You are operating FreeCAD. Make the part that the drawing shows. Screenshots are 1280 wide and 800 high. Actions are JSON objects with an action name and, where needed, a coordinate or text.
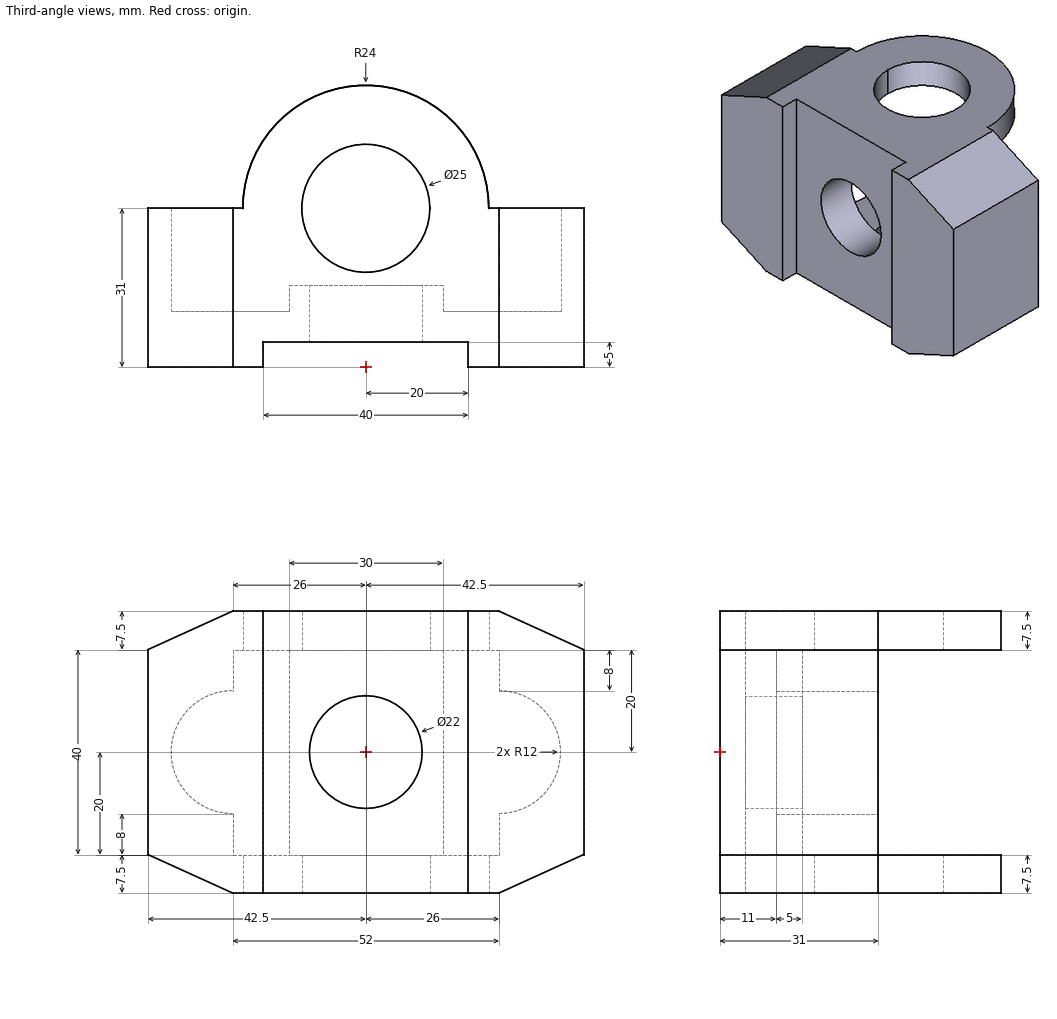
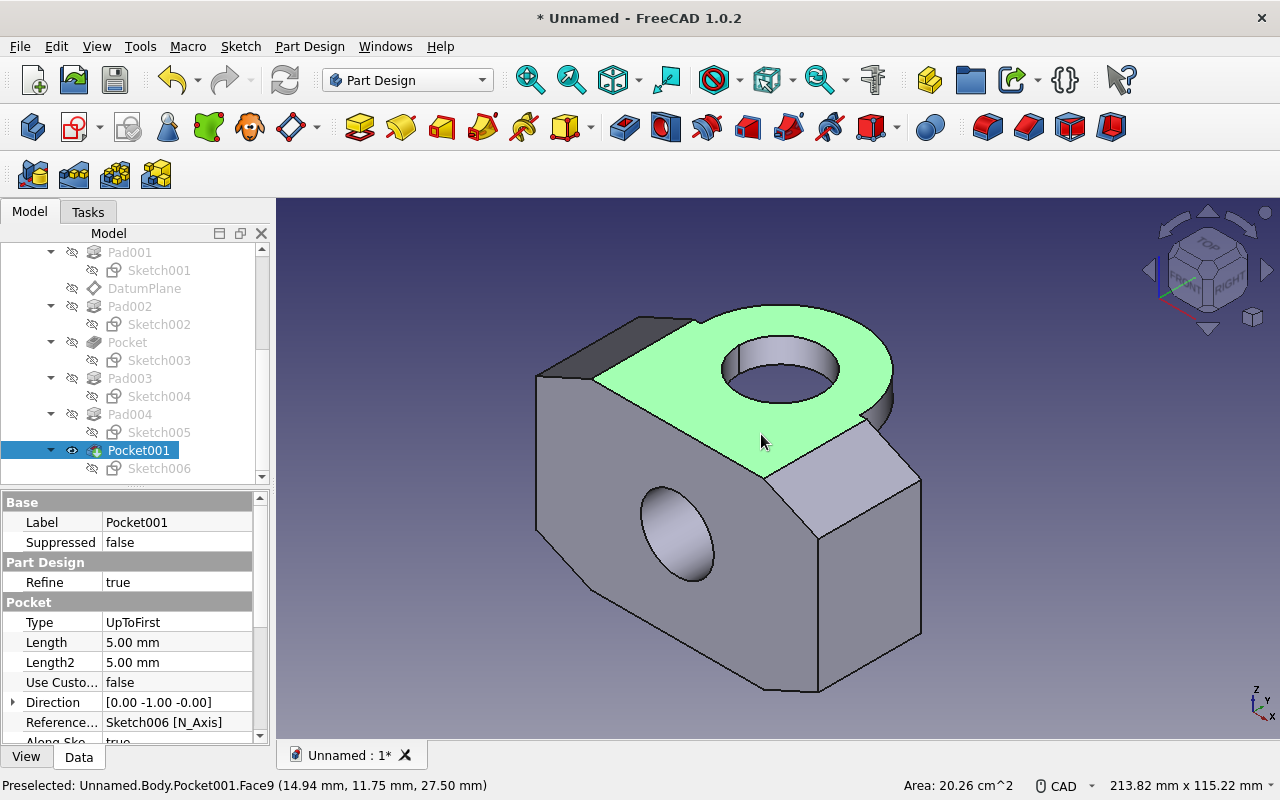
{"action": "left_click", "coordinate": [74, 128]}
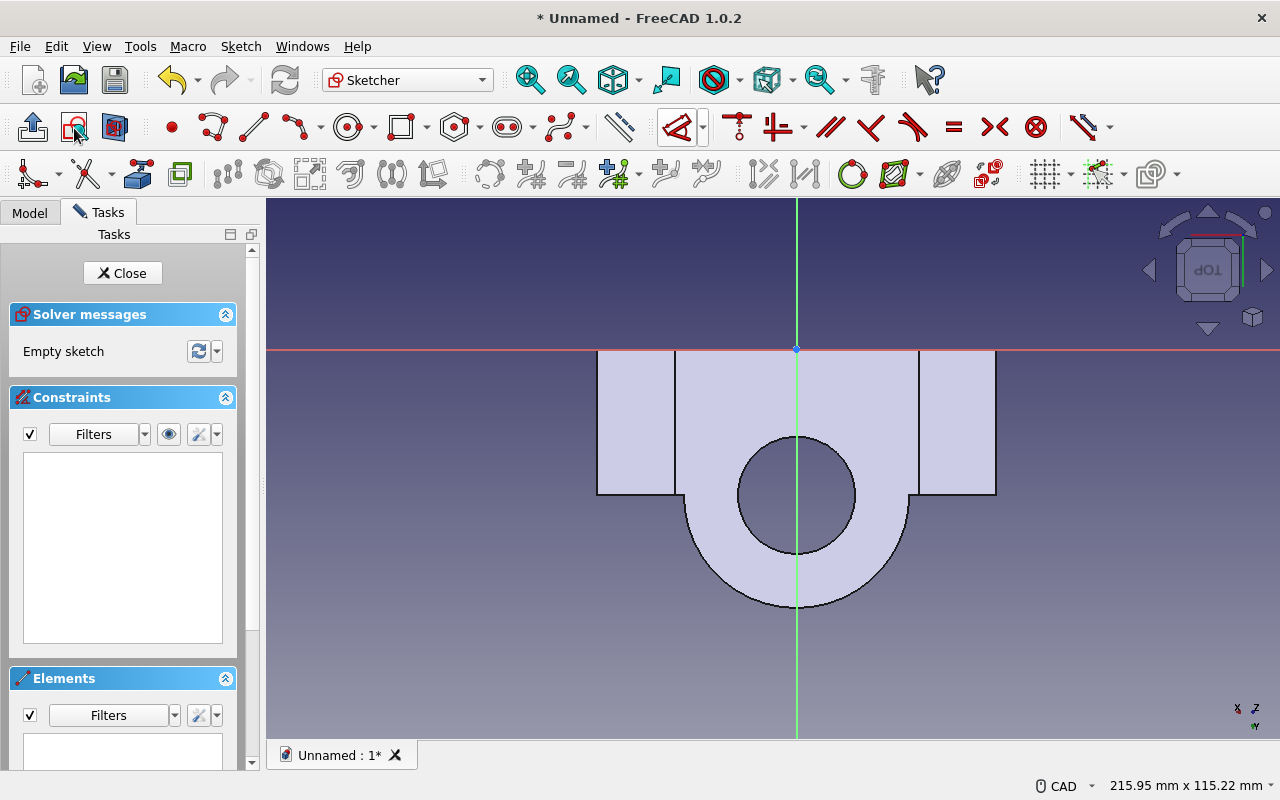
{"action": "scroll", "coordinate": [836, 315], "scroll_direction": "up", "scroll_amount": 6}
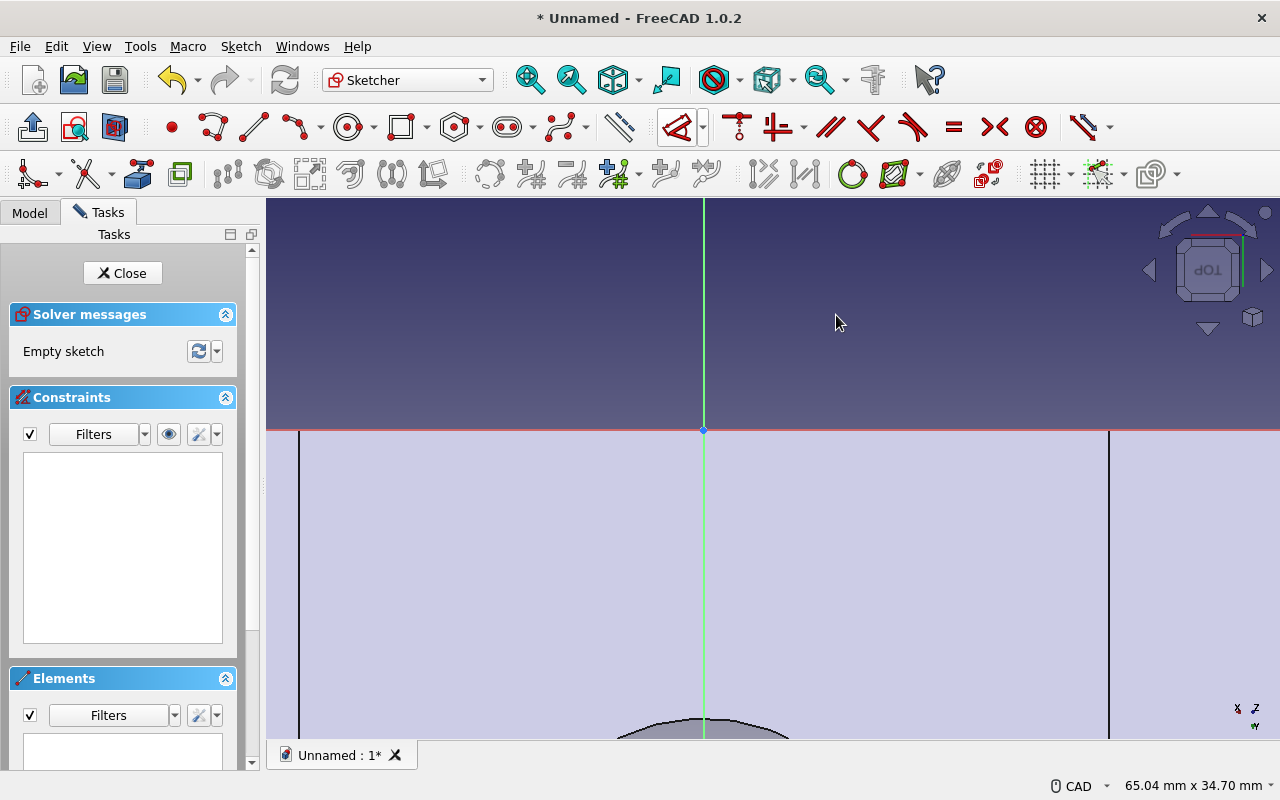
{"action": "left_click", "coordinate": [400, 128]}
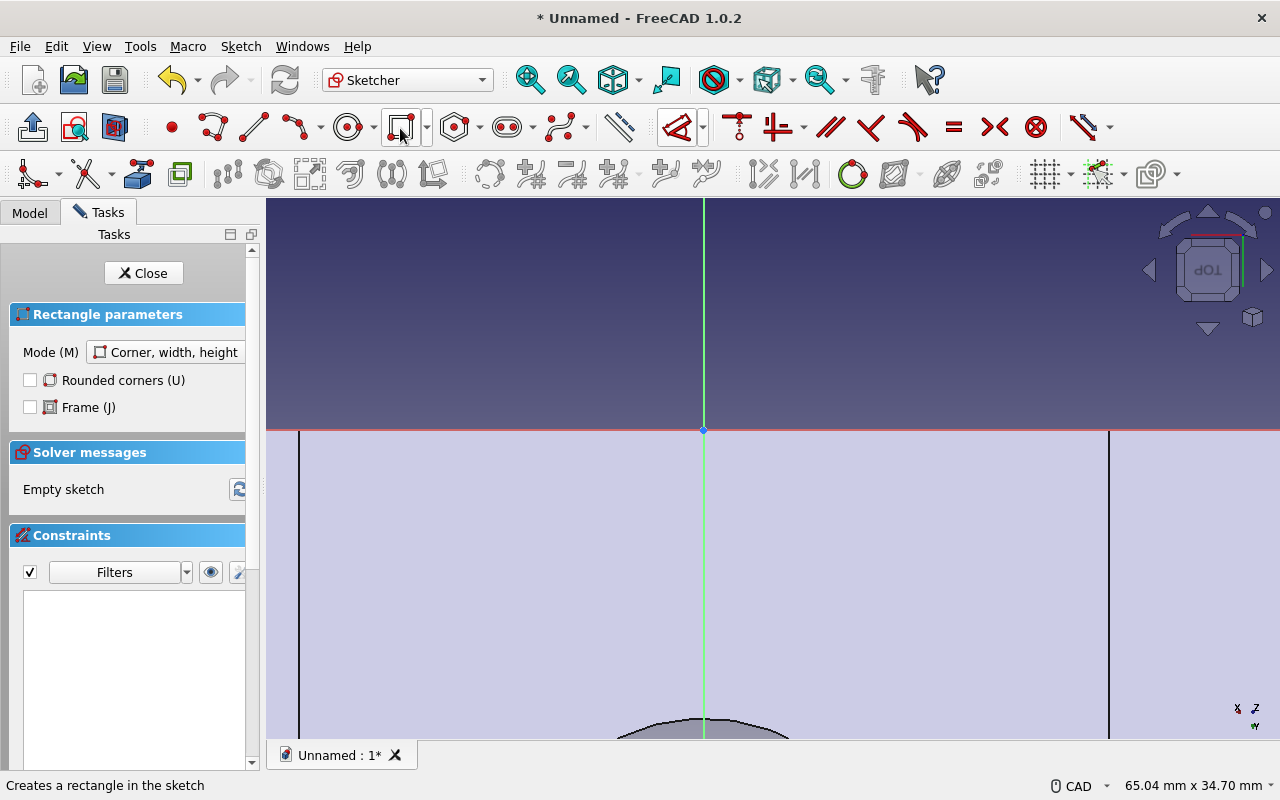
{"action": "left_click", "coordinate": [392, 430]}
{"action": "left_click", "coordinate": [1016, 508]}
{"action": "key", "text": "Escape"}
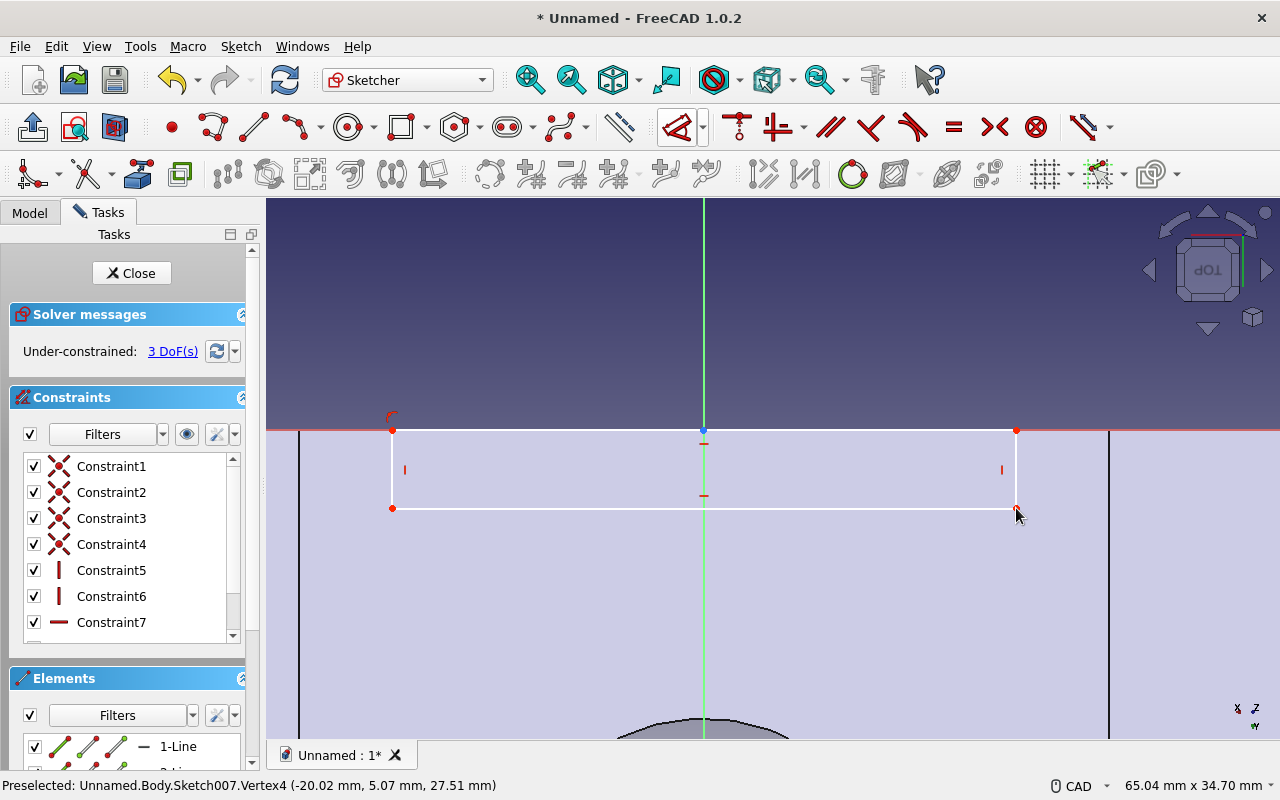
{"action": "left_click", "coordinate": [392, 454]}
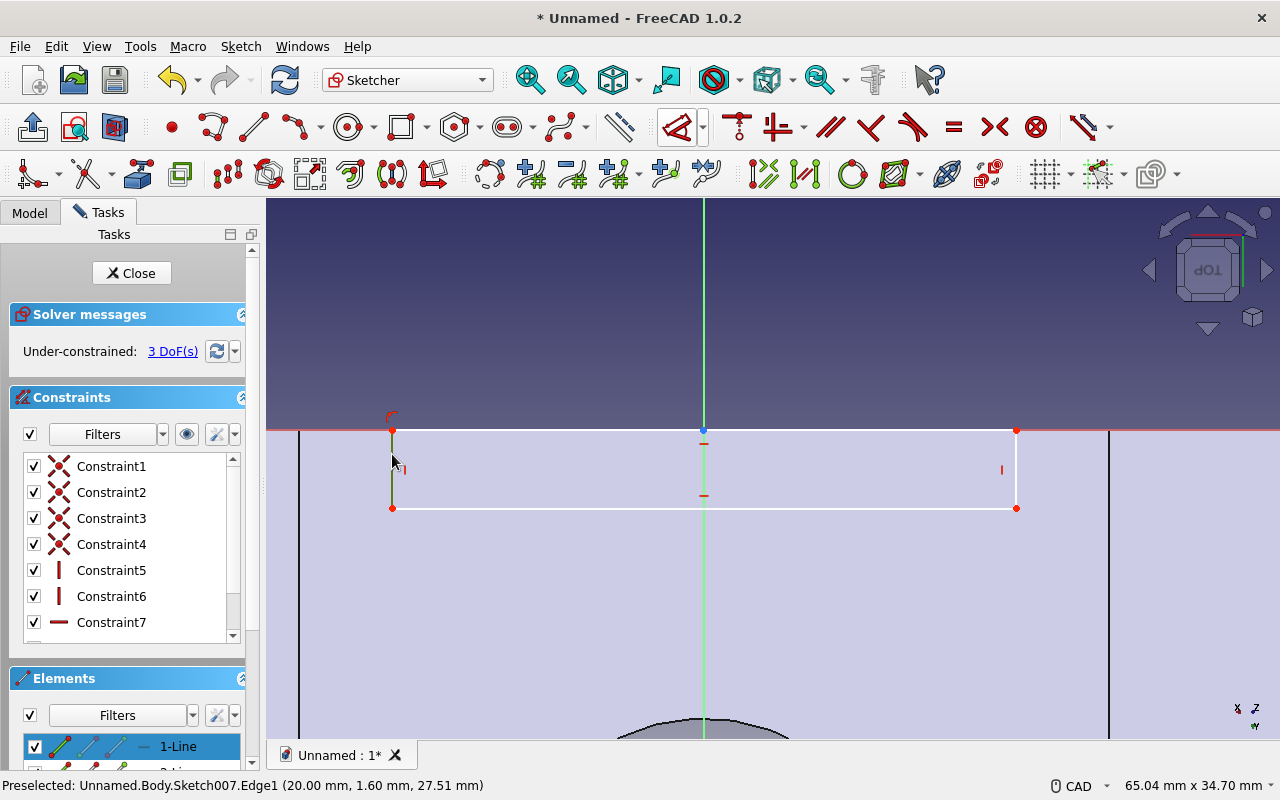
{"action": "key", "text": "i"}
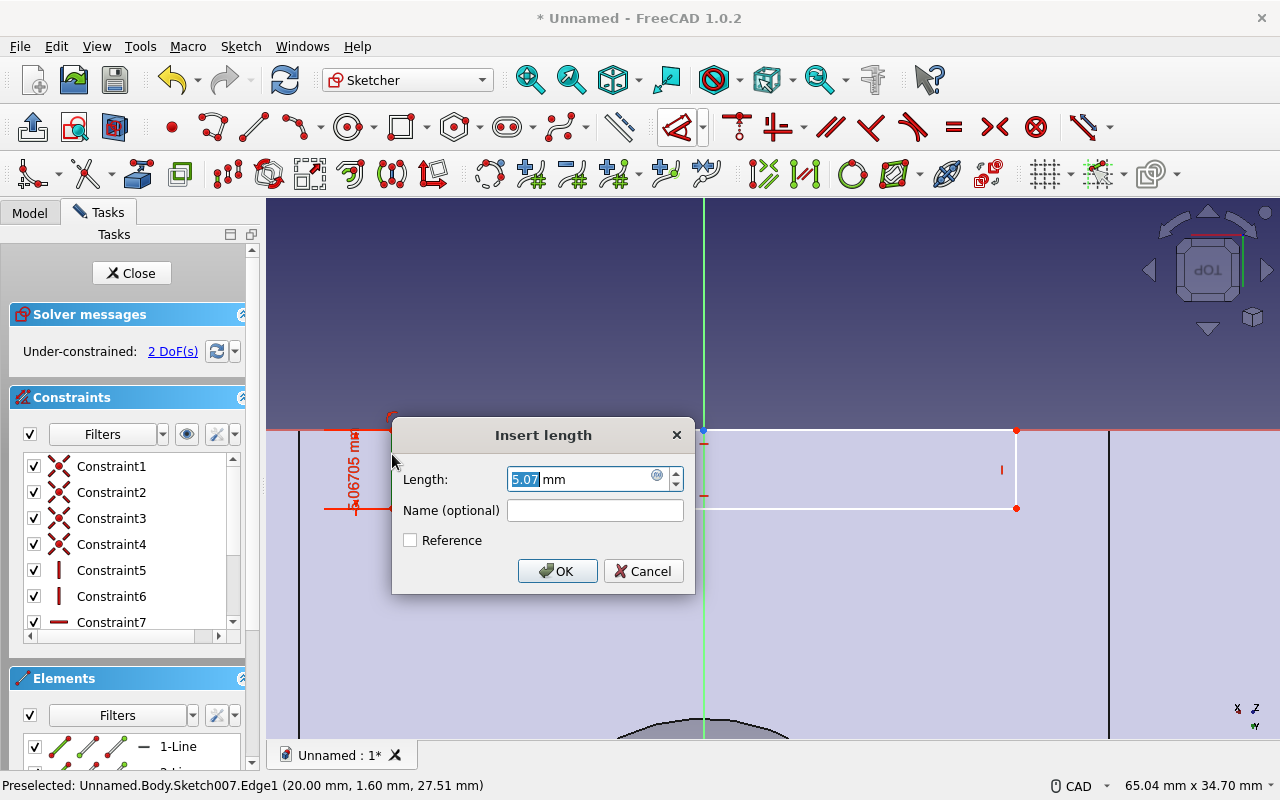
{"action": "type", "text": "5"}
{"action": "key", "text": "Return"}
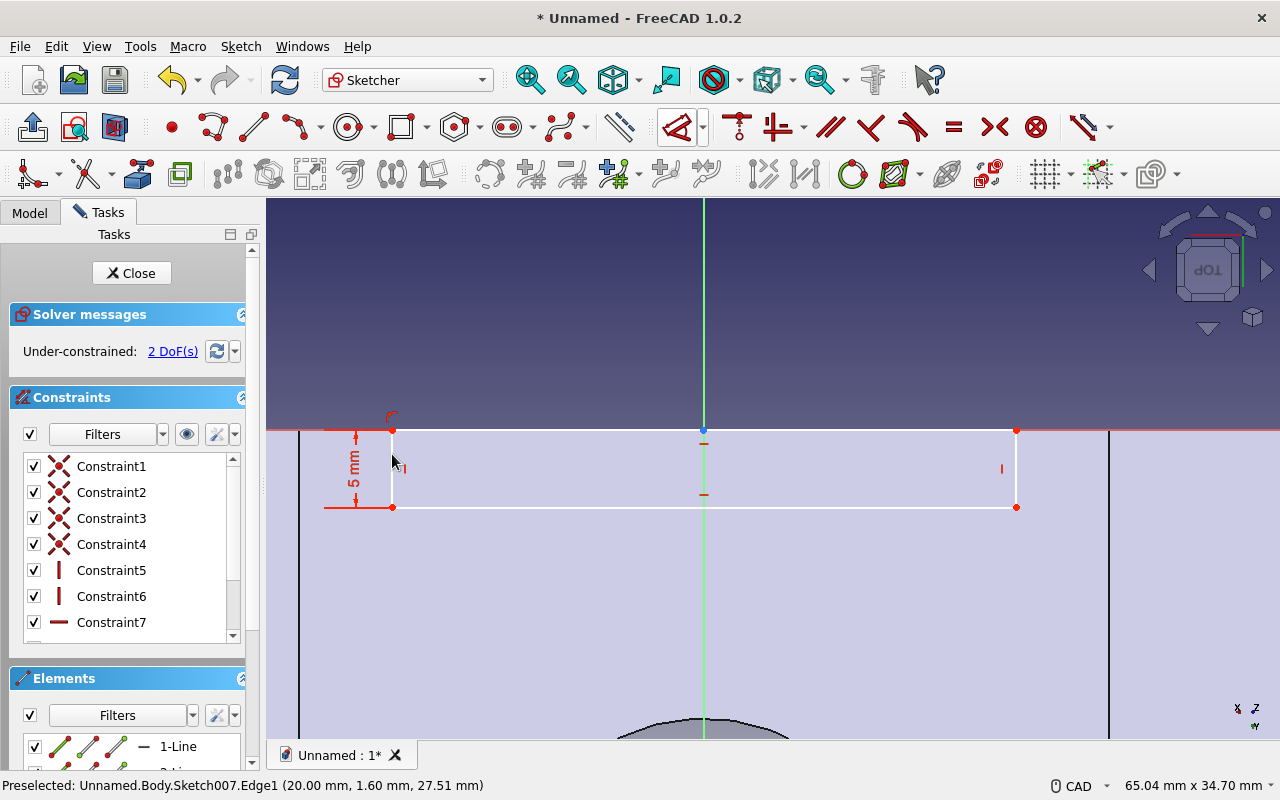
{"action": "left_click", "coordinate": [579, 508]}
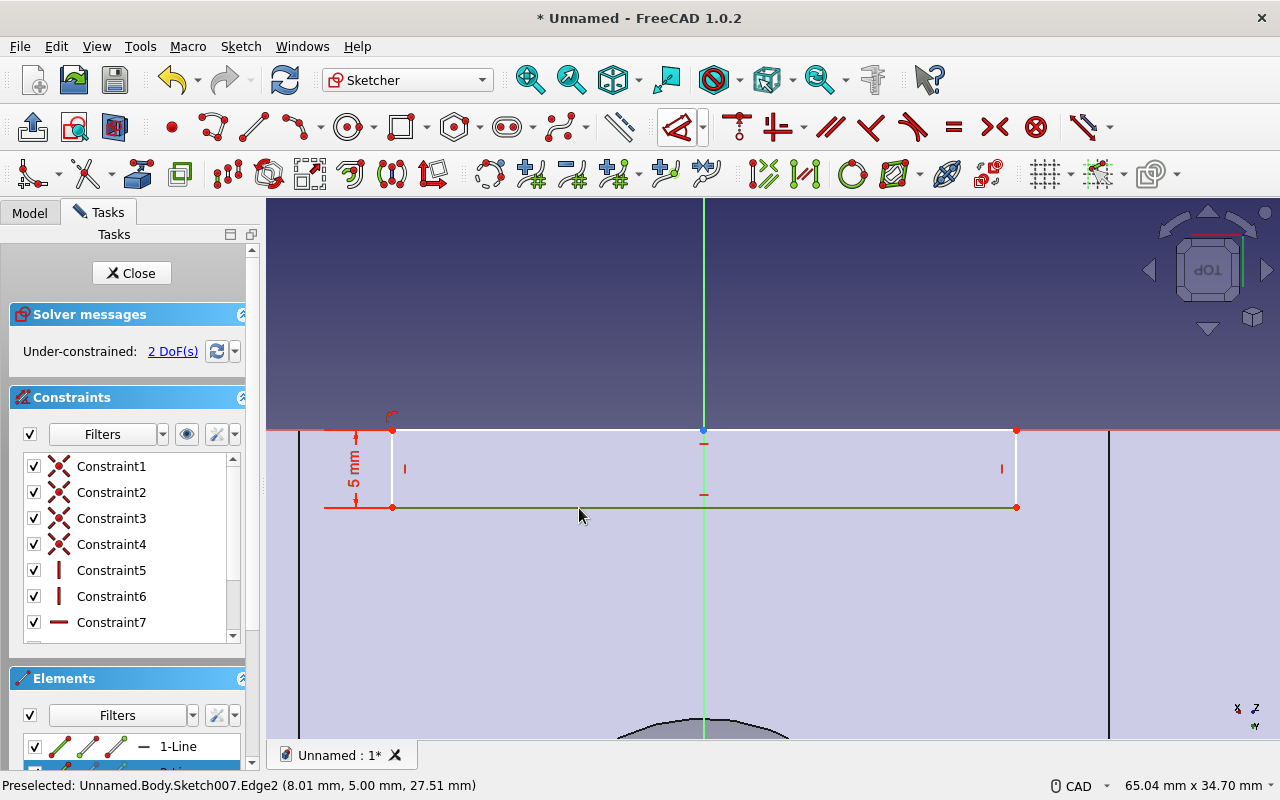
{"action": "left_click", "coordinate": [702, 128]}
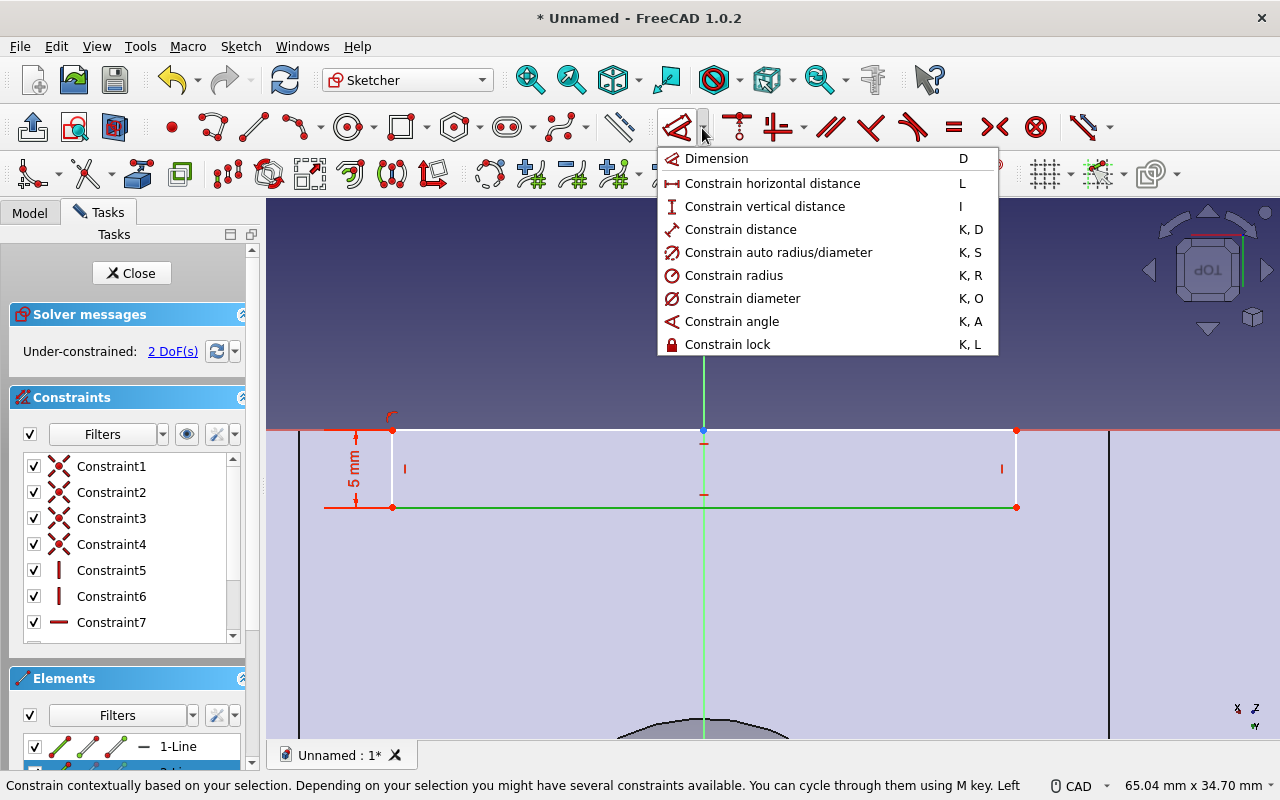
{"action": "left_click", "coordinate": [828, 184]}